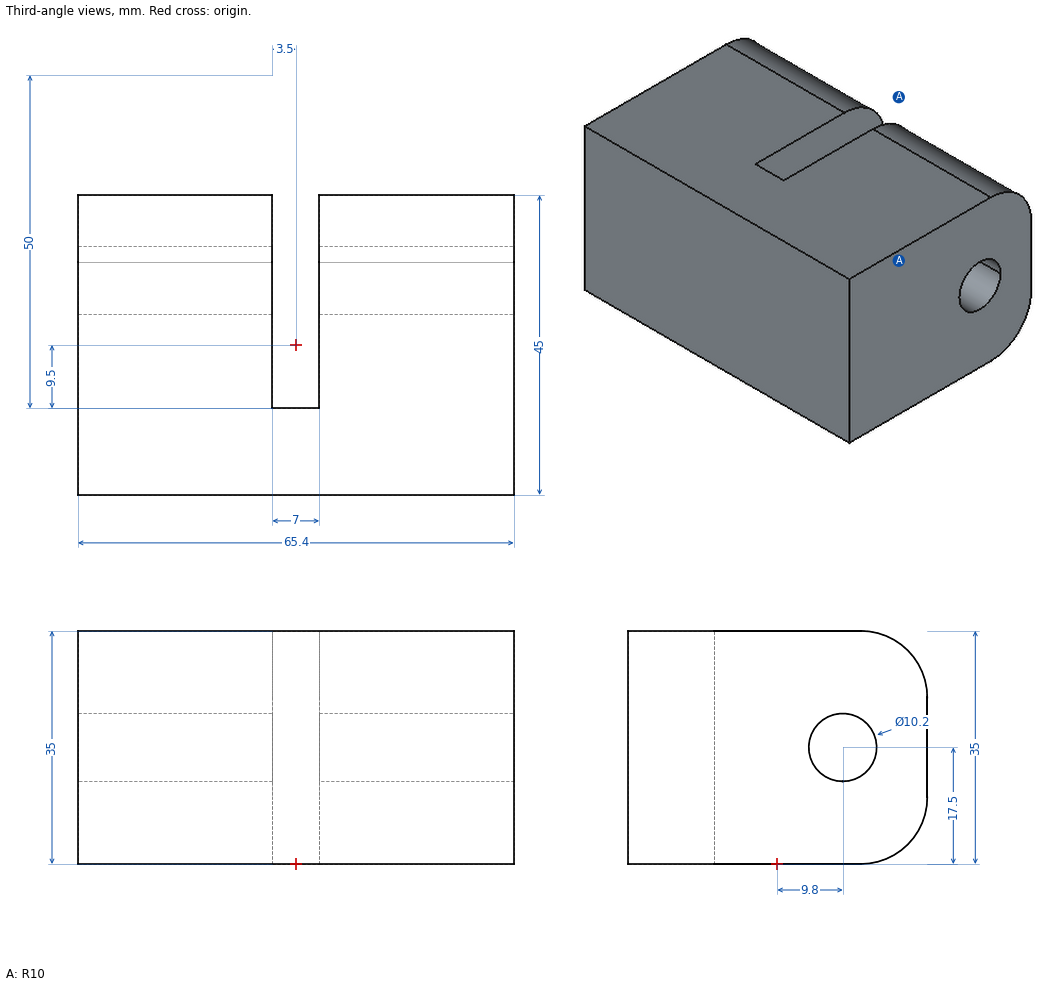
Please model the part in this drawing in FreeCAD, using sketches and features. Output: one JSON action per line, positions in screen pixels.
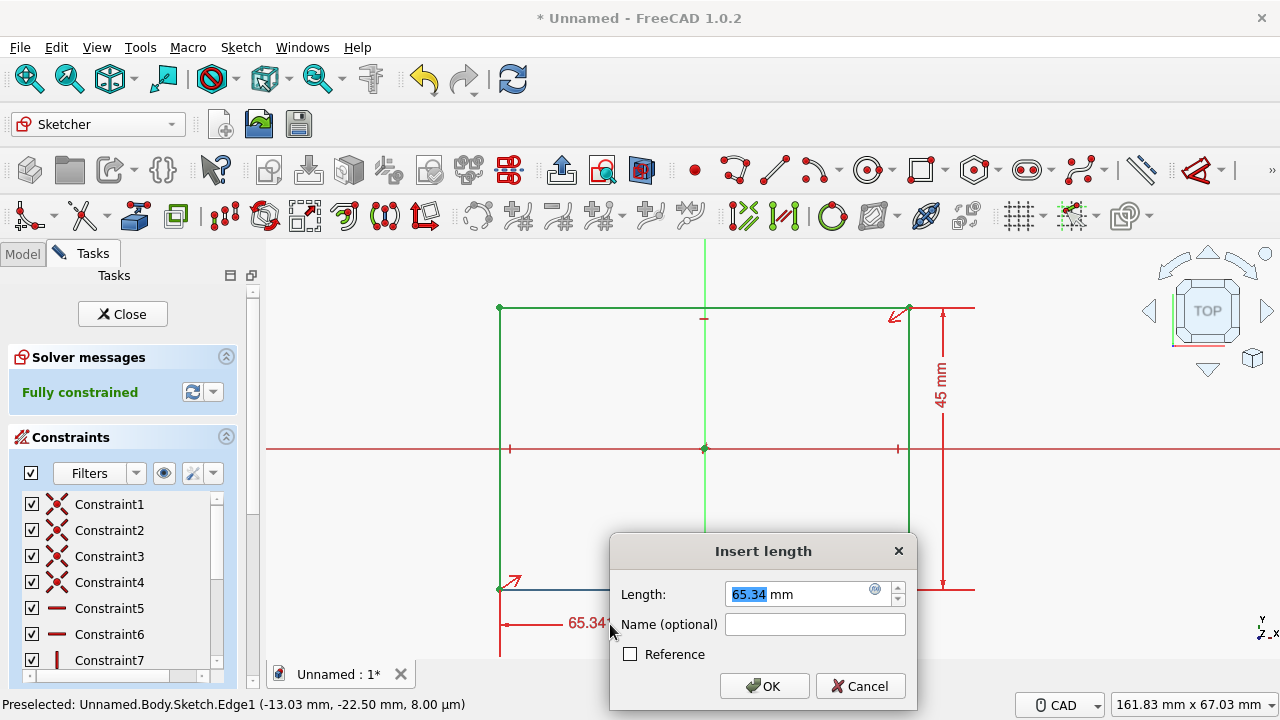
{"action": "type", "text": "65.4"}
{"action": "key", "text": "Return"}
{"action": "key", "text": "Escape"}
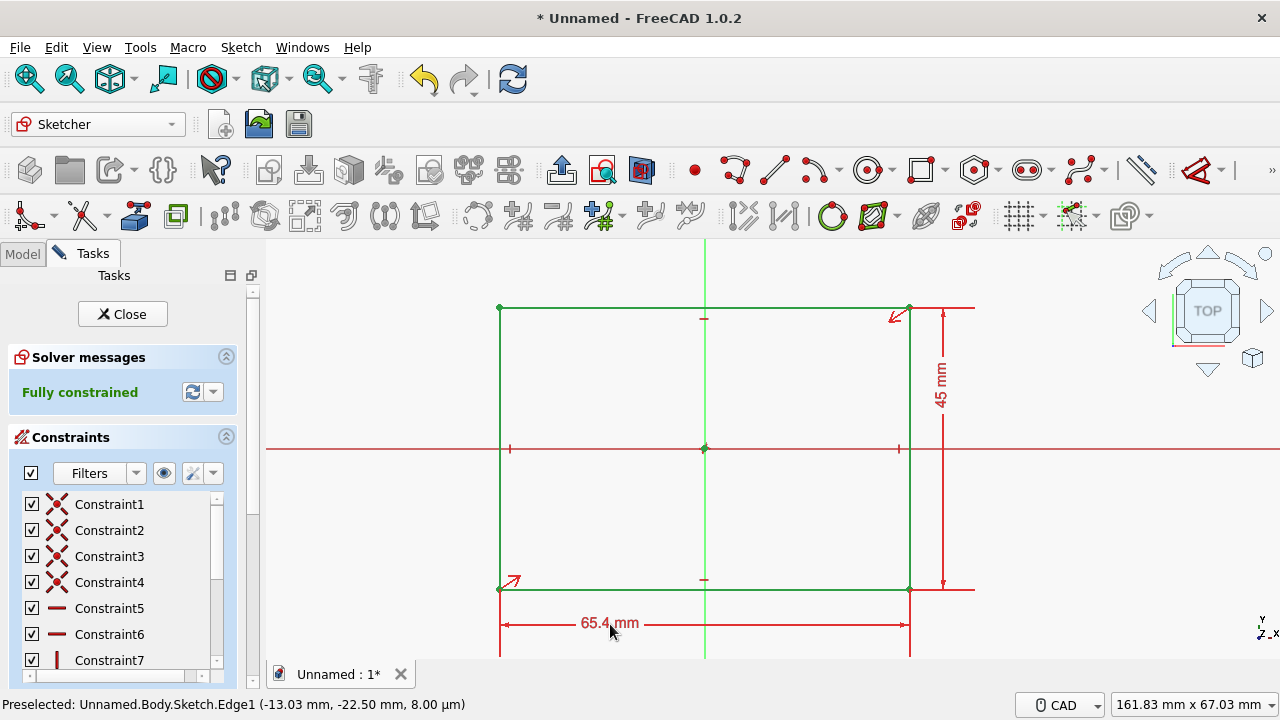
{"action": "left_click", "coordinate": [123, 314]}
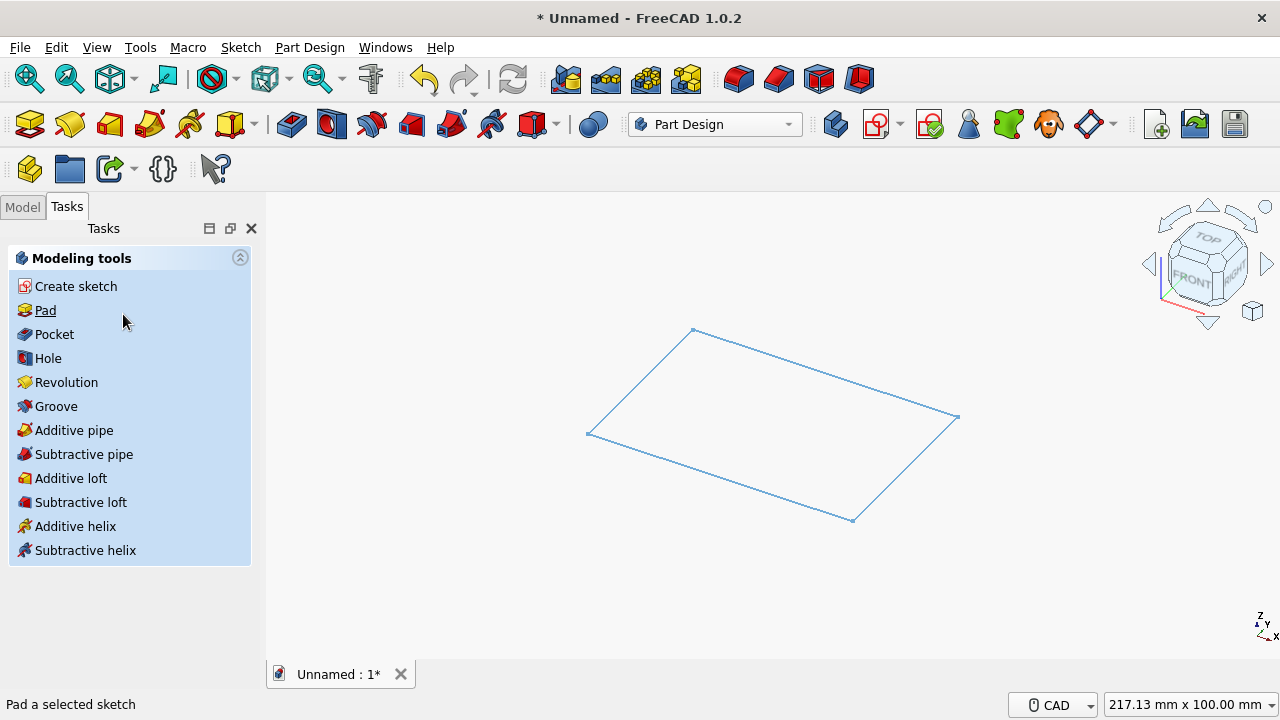
{"action": "left_click", "coordinate": [30, 124]}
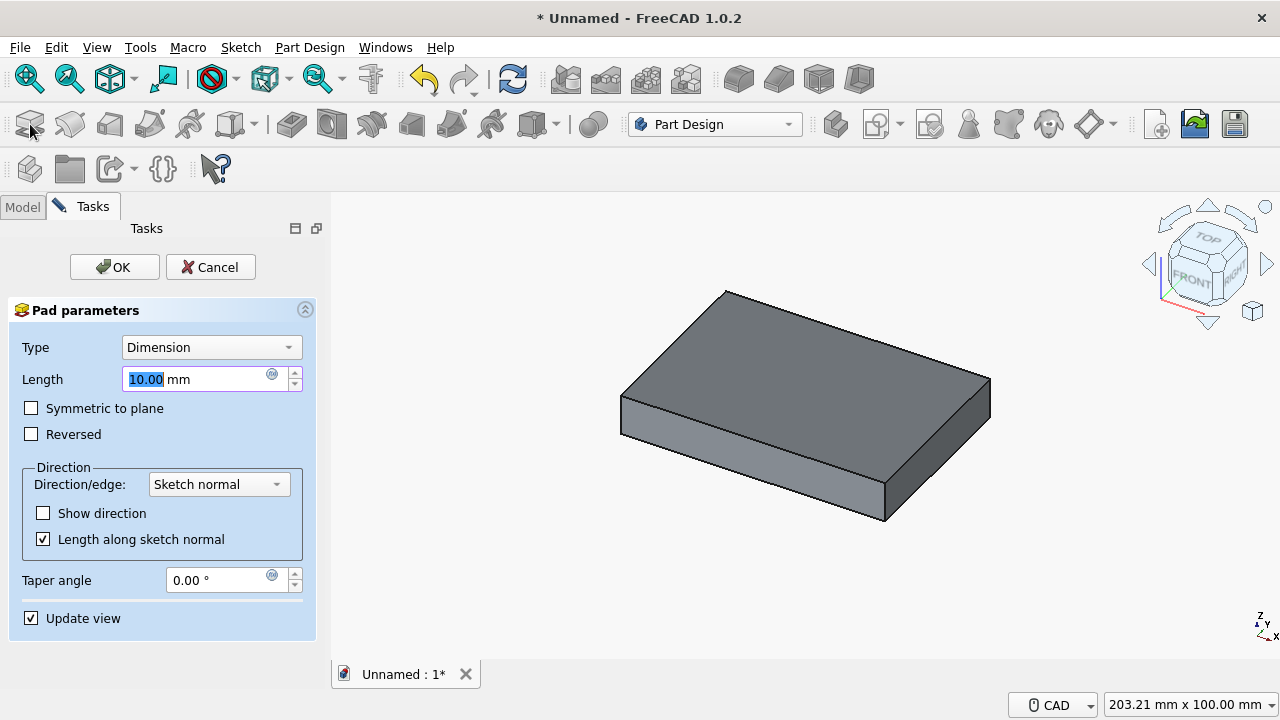
{"action": "type", "text": "35"}
{"action": "key", "text": "Tab"}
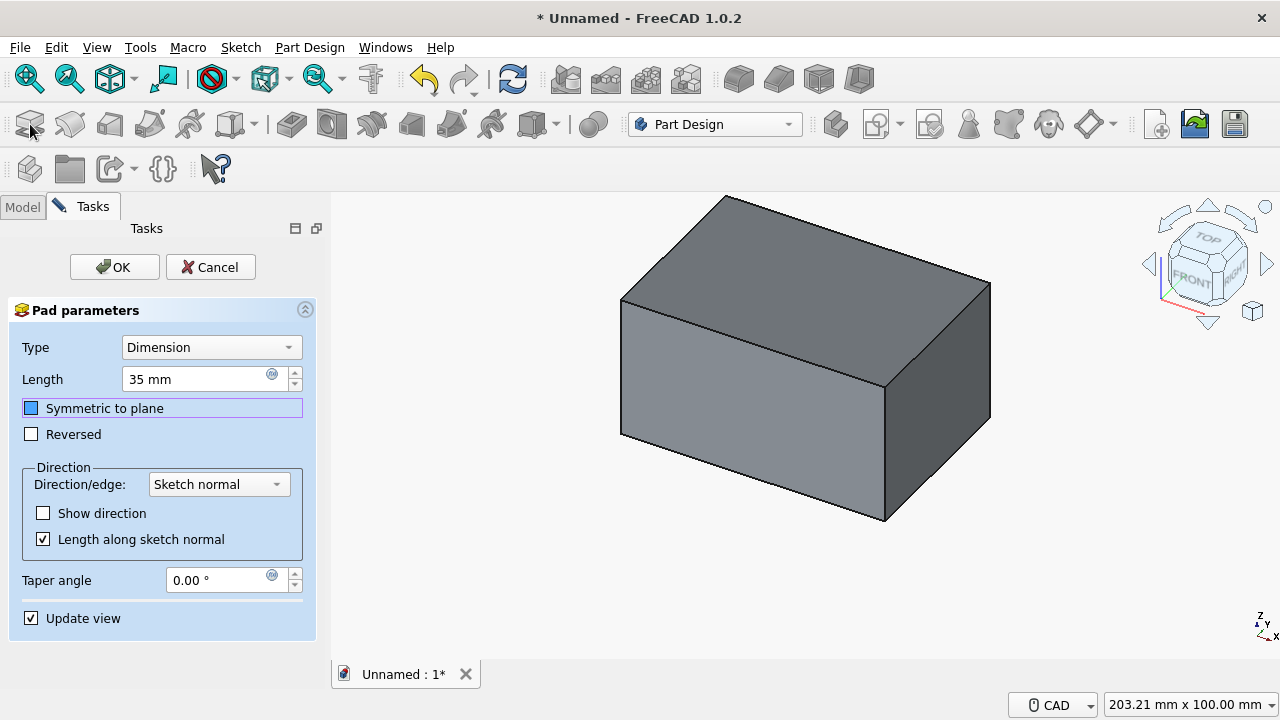
{"action": "left_click", "coordinate": [115, 267]}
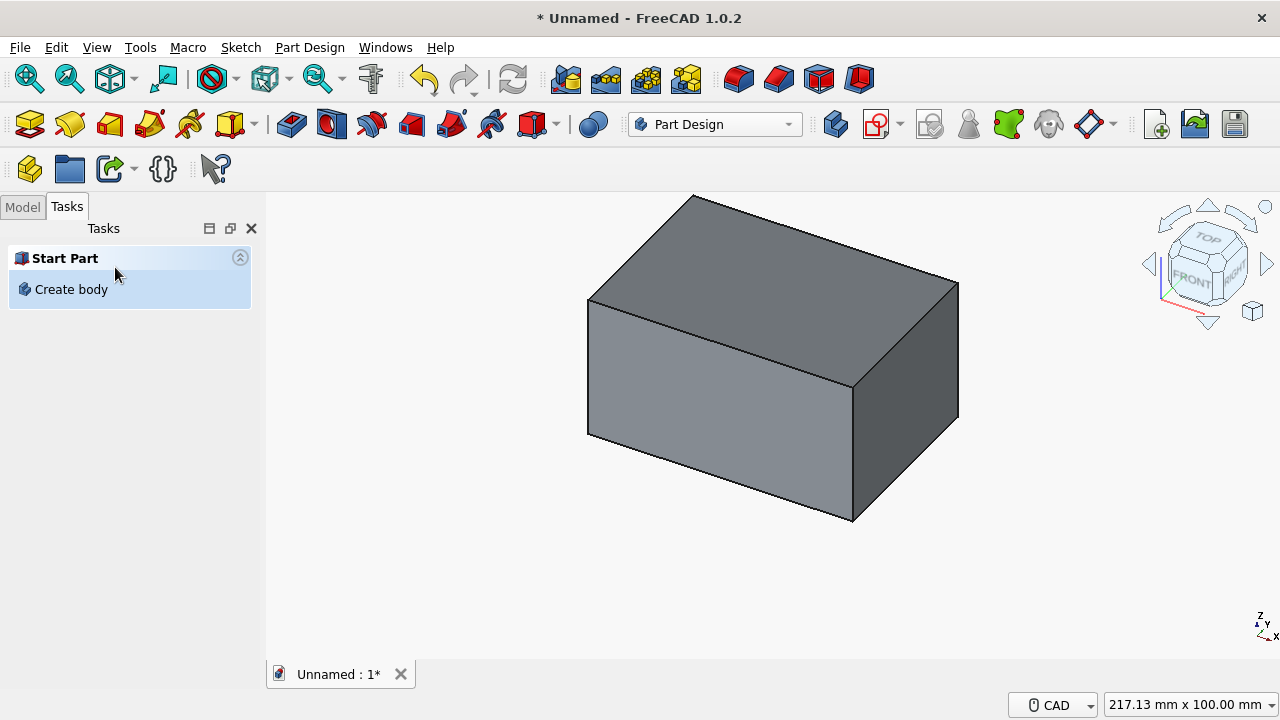
{"action": "key", "text": "0"}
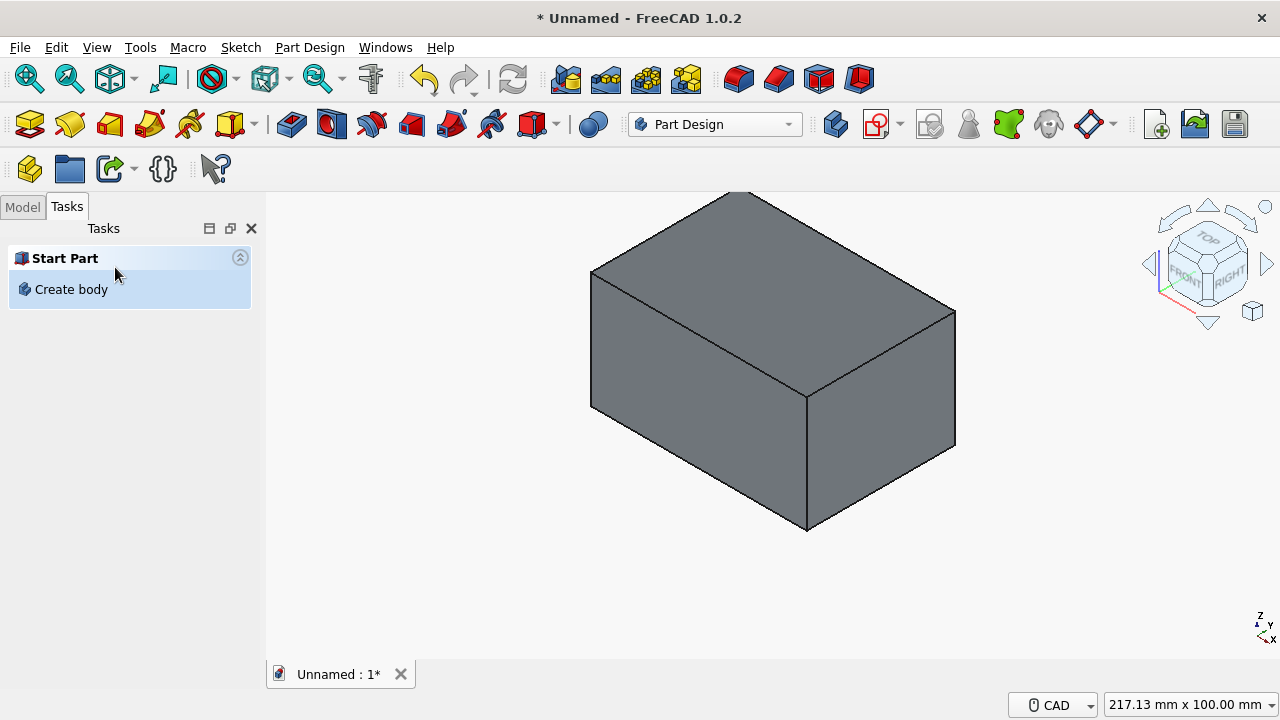
{"action": "left_click", "coordinate": [30, 80]}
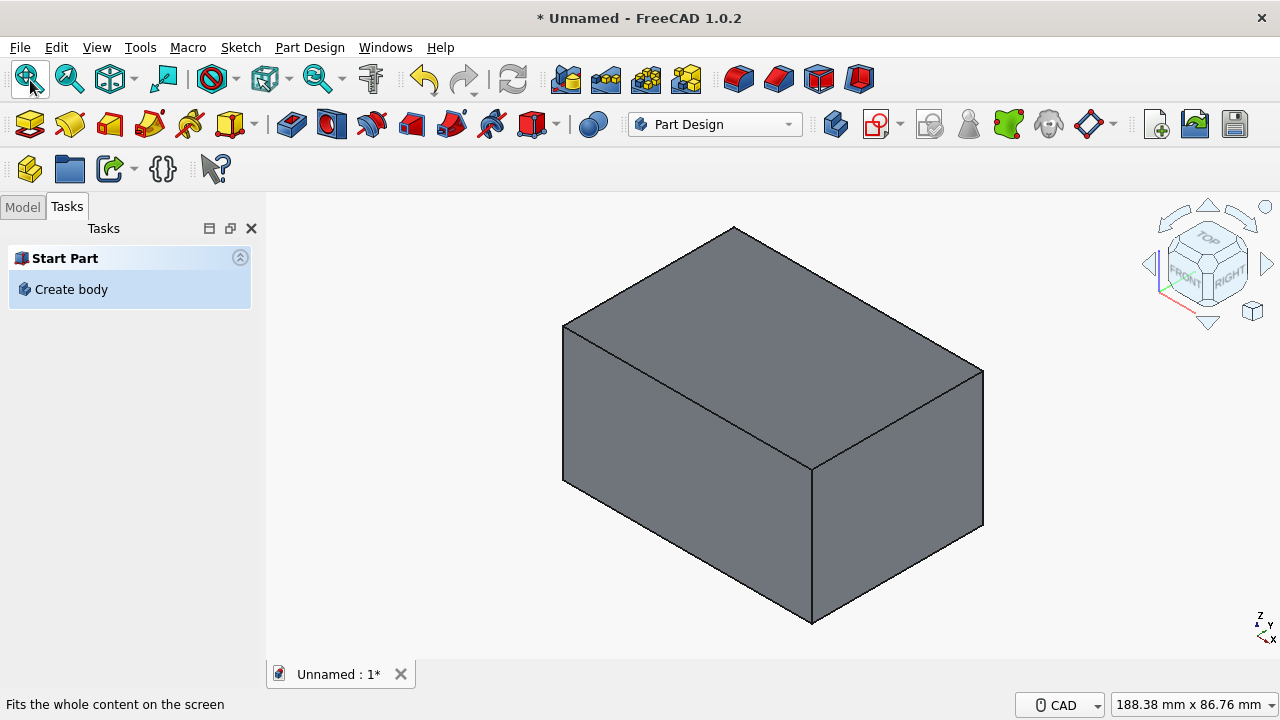
{"action": "key", "text": "2"}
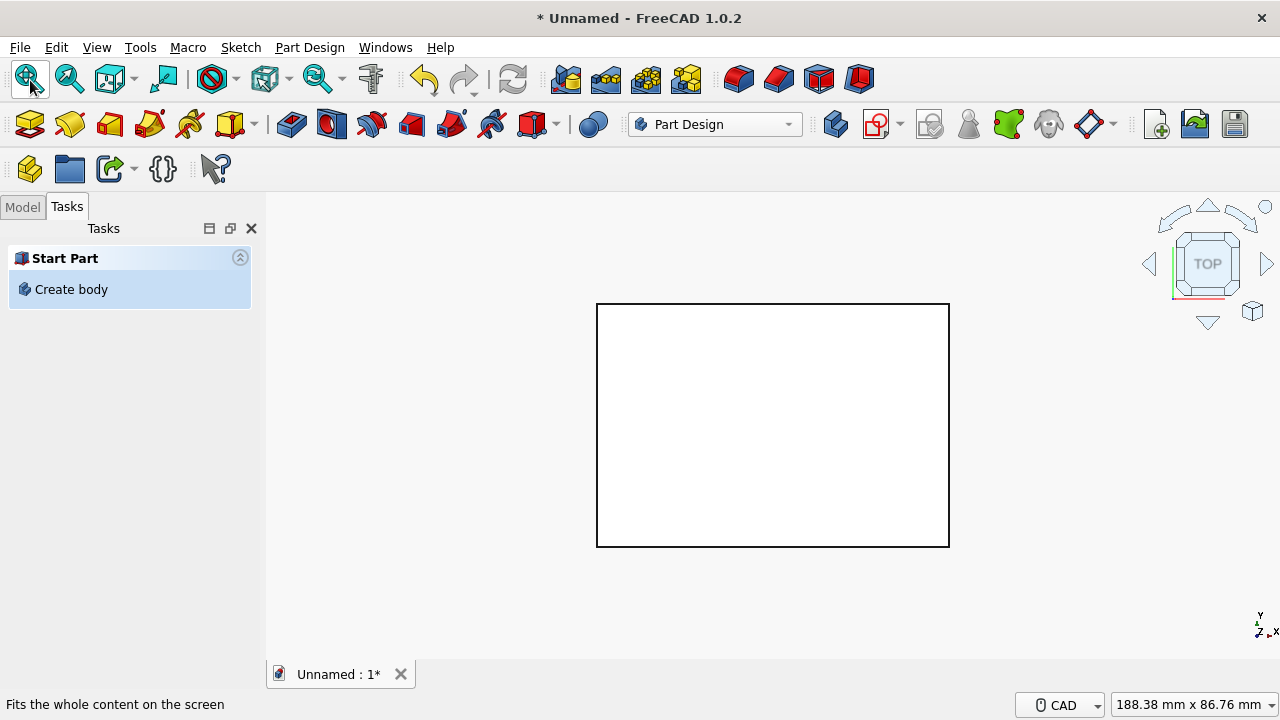
{"action": "left_click", "coordinate": [773, 303]}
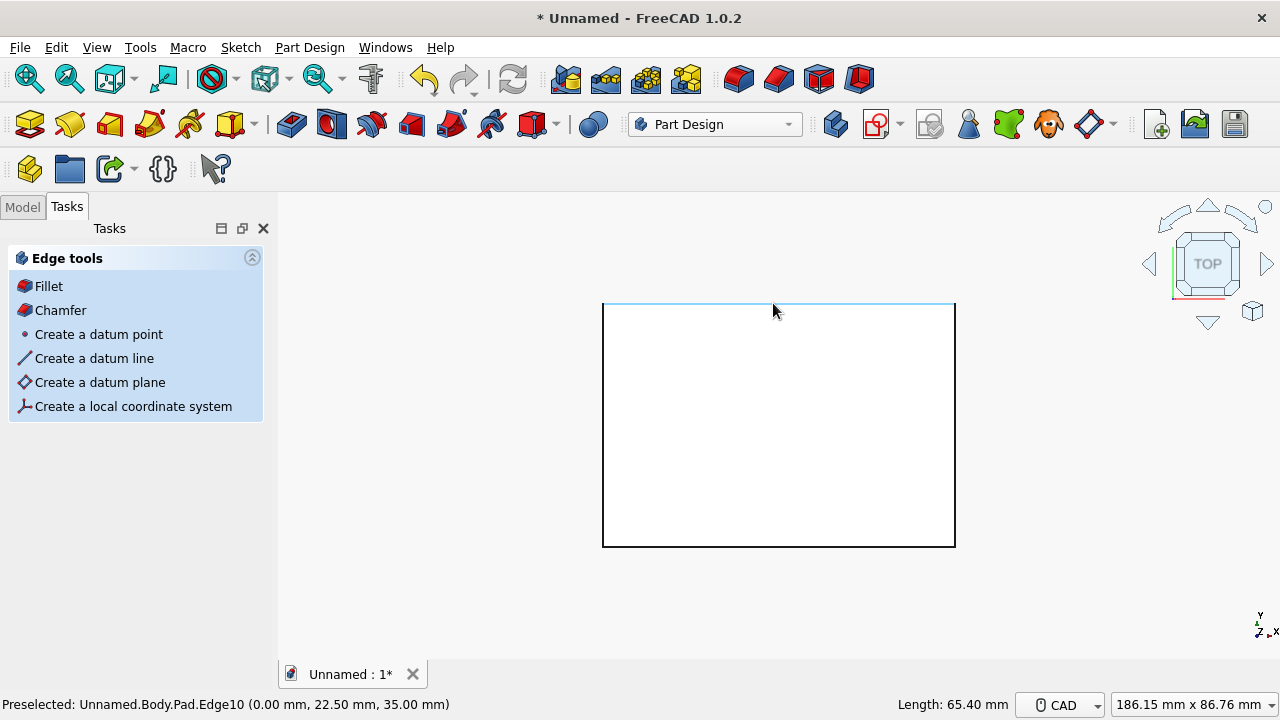
{"action": "key", "text": "1"}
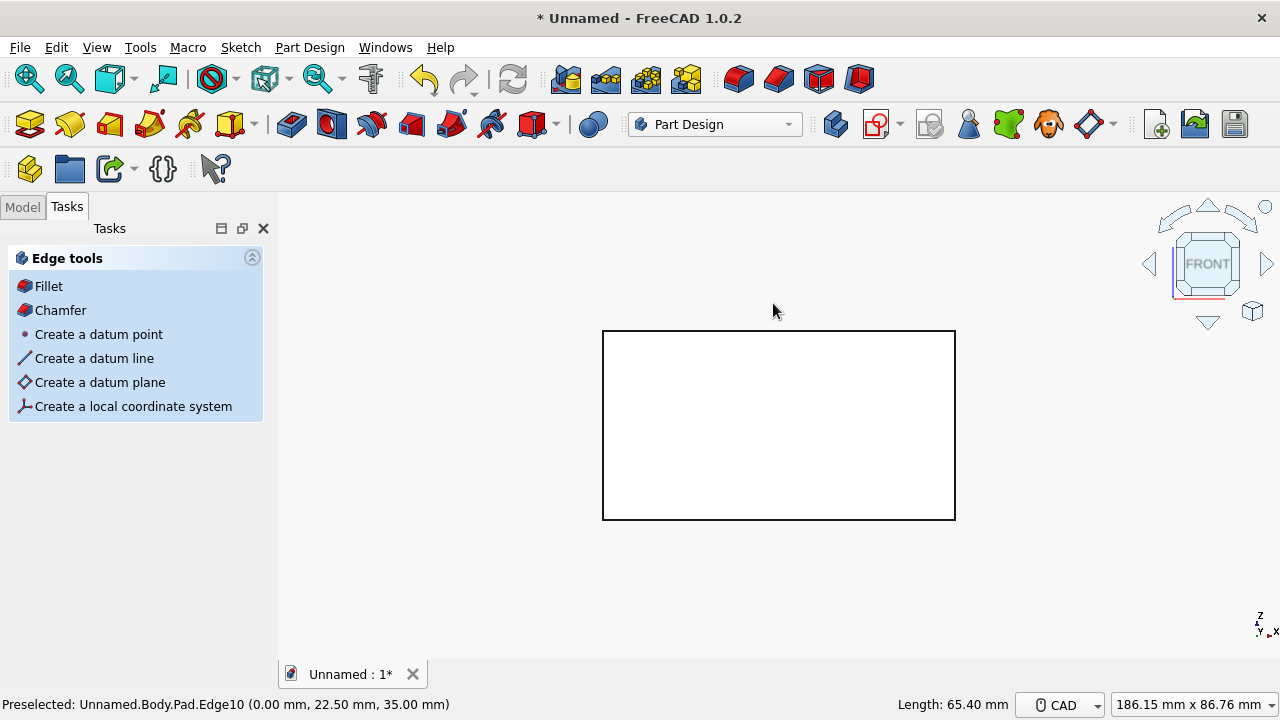
{"action": "left_click", "coordinate": [30, 80]}